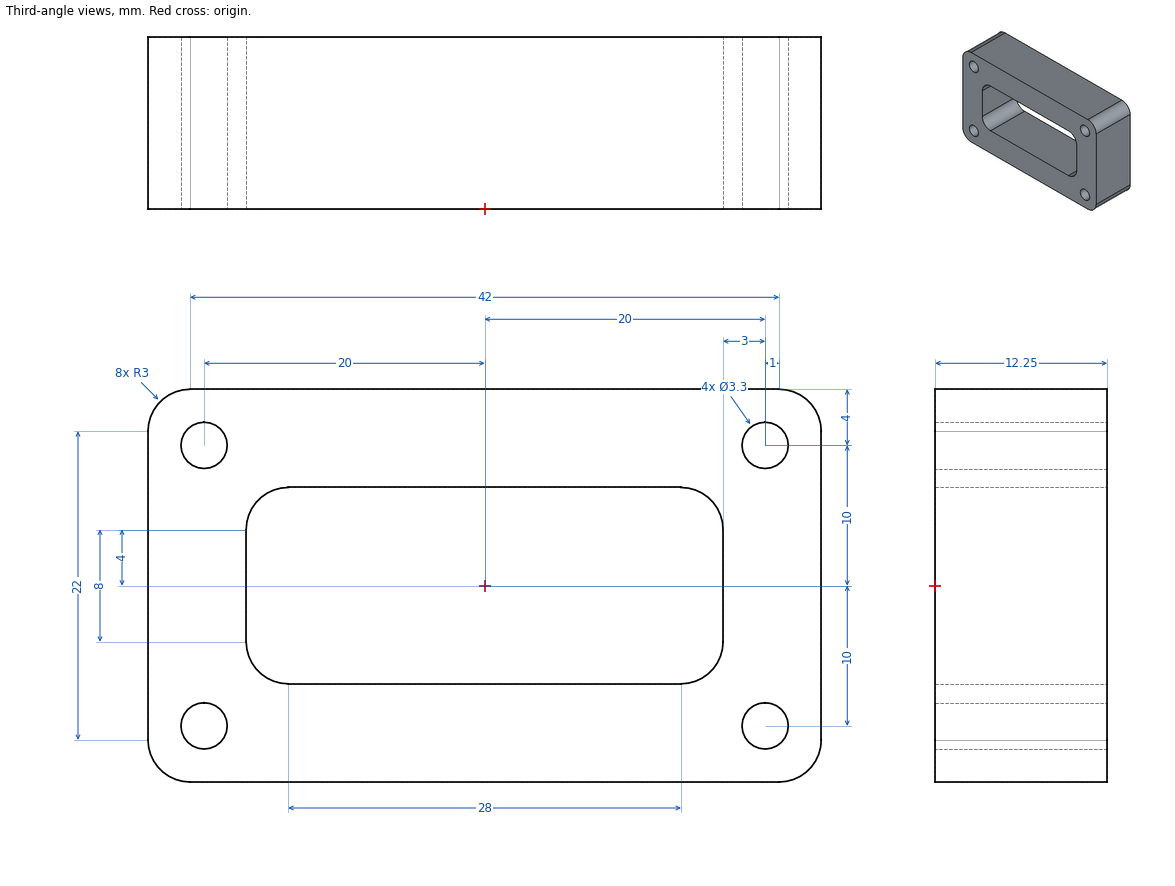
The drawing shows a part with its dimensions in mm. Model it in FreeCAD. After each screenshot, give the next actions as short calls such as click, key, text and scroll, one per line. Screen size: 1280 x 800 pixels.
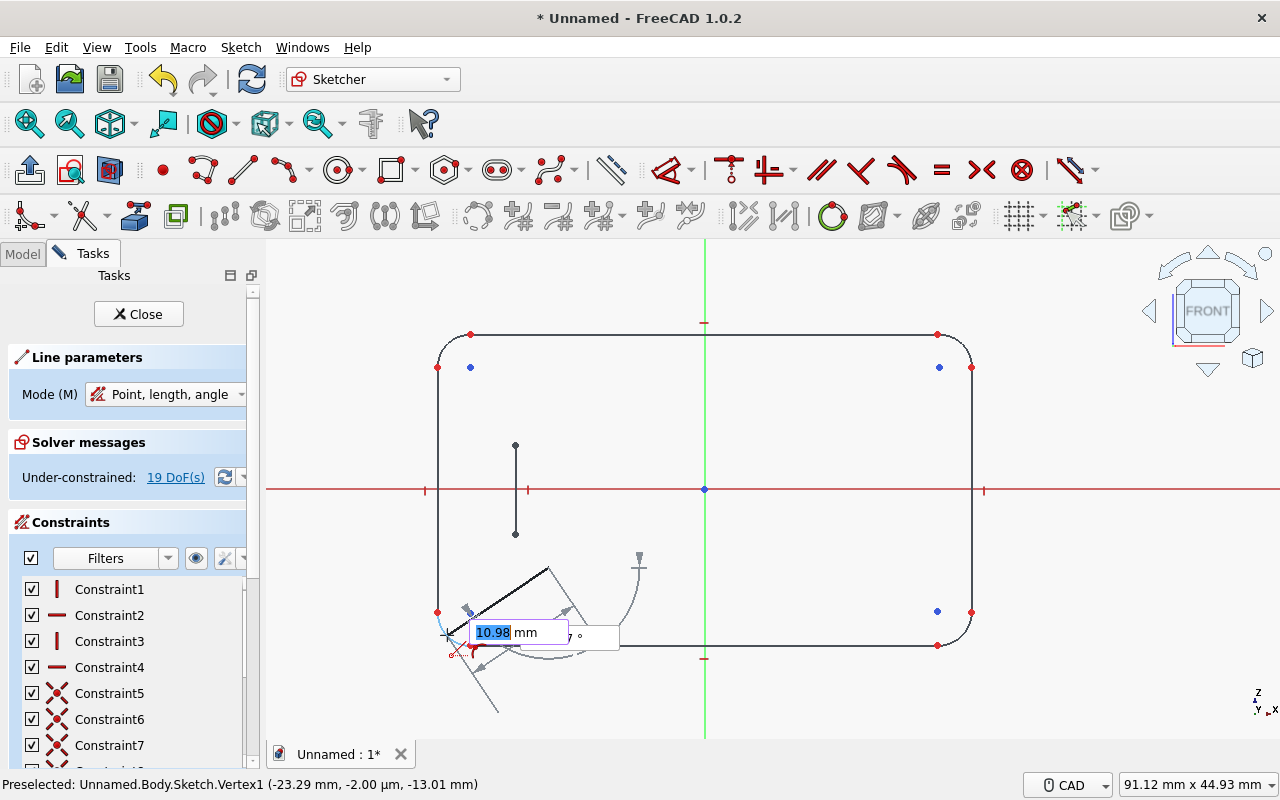
click(860, 567)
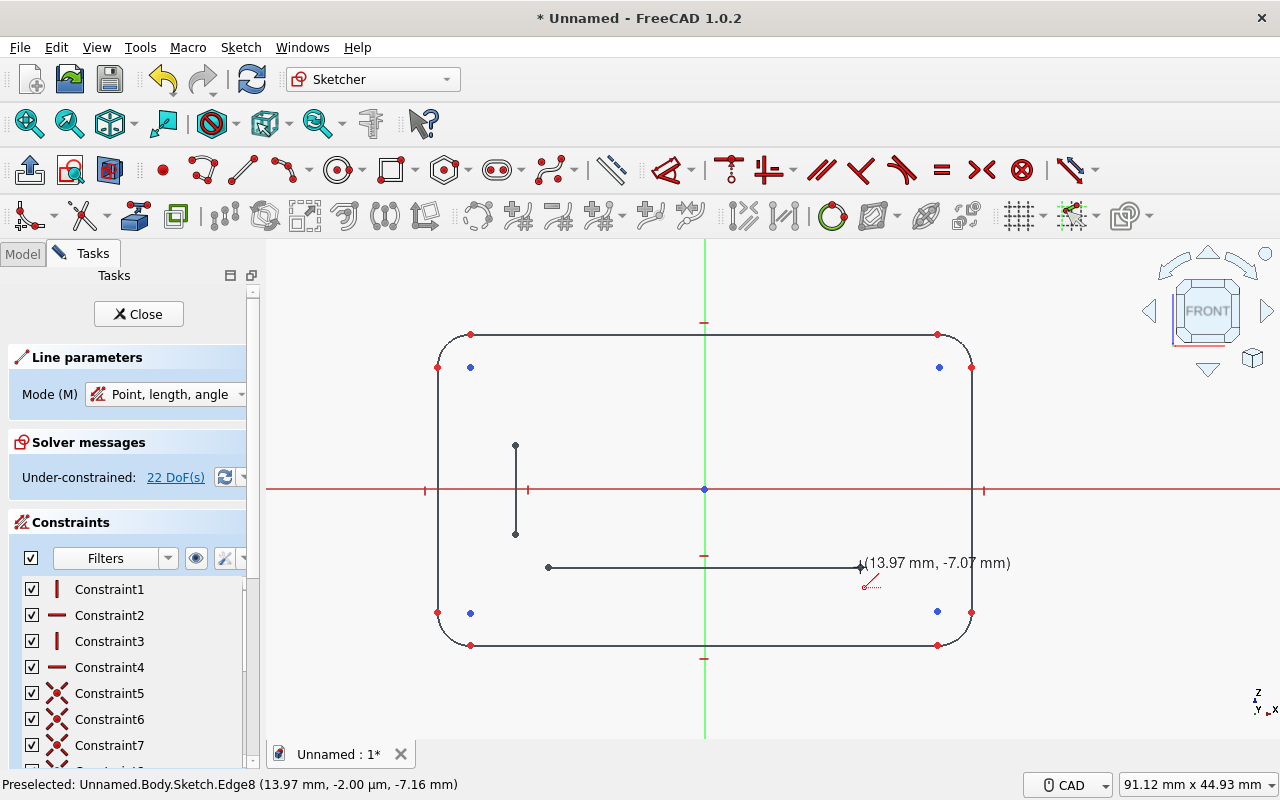
click(894, 534)
click(894, 445)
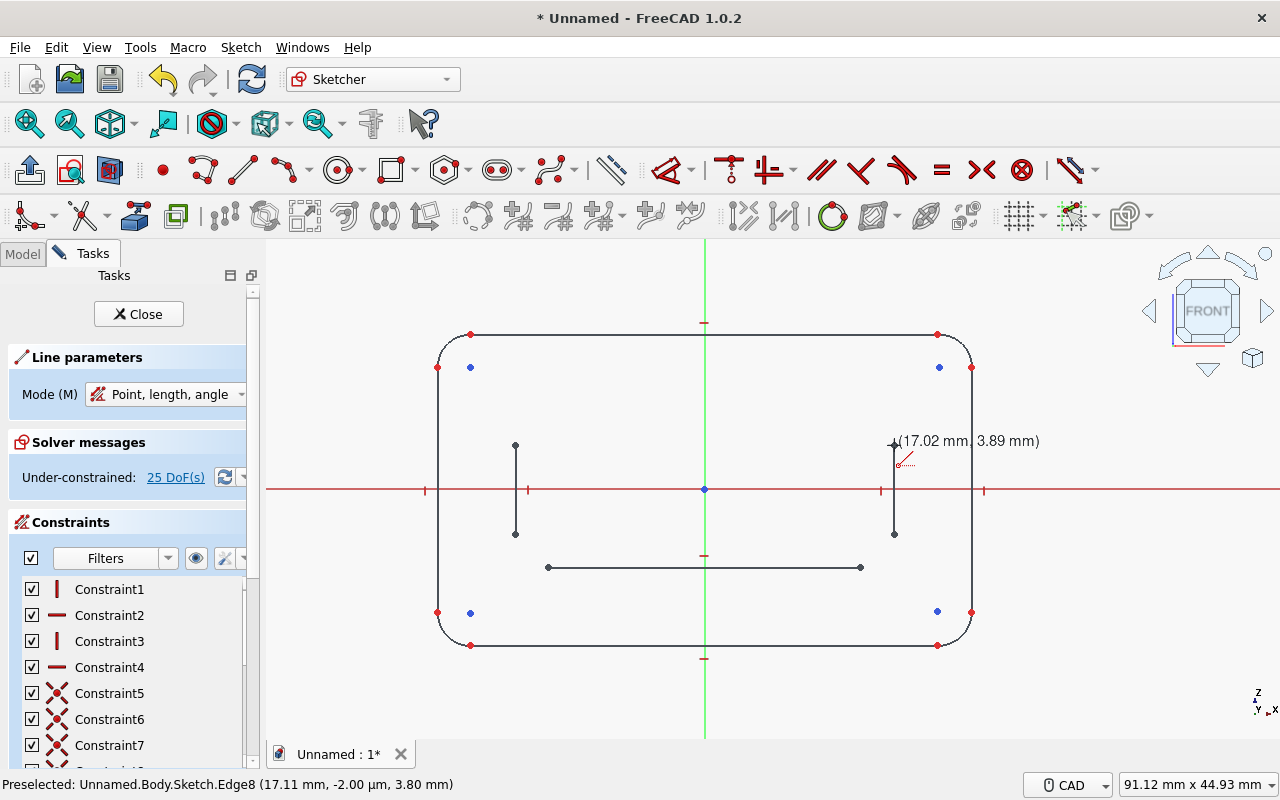
click(860, 411)
click(549, 411)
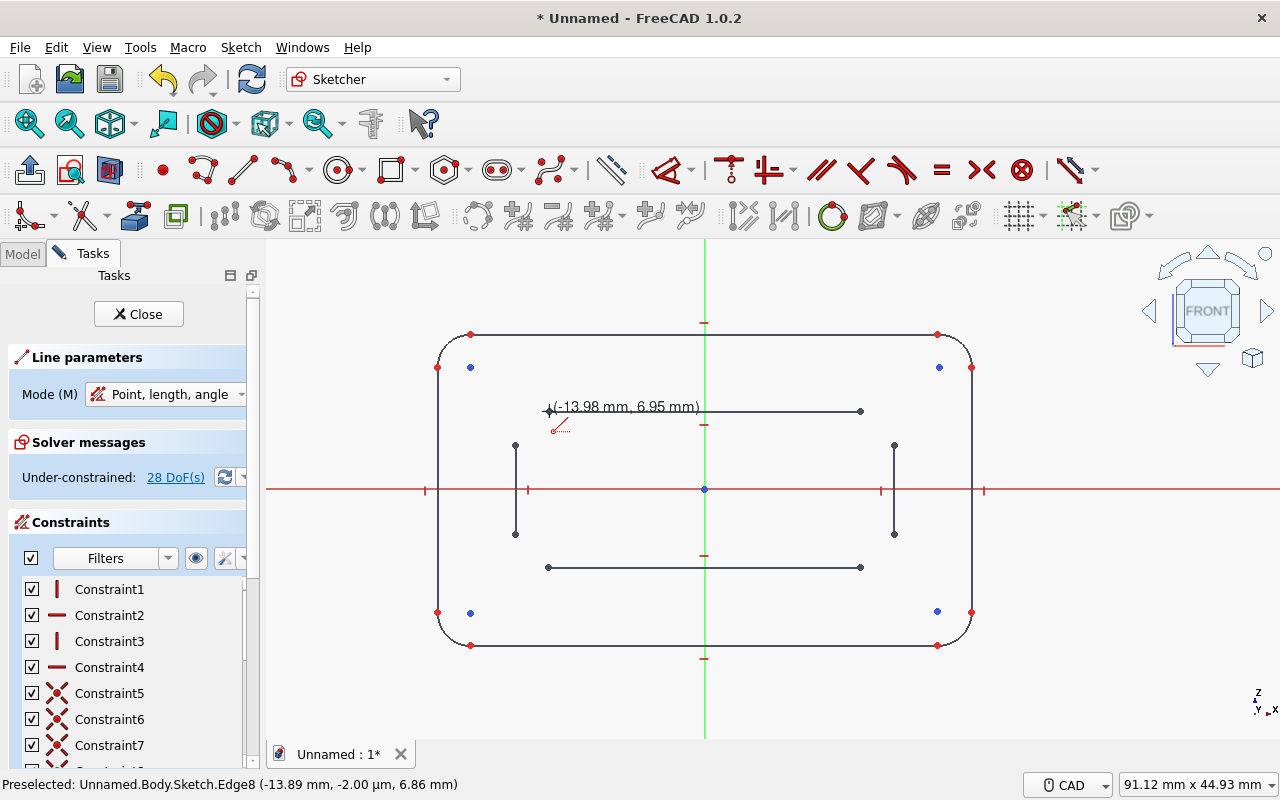
click(284, 170)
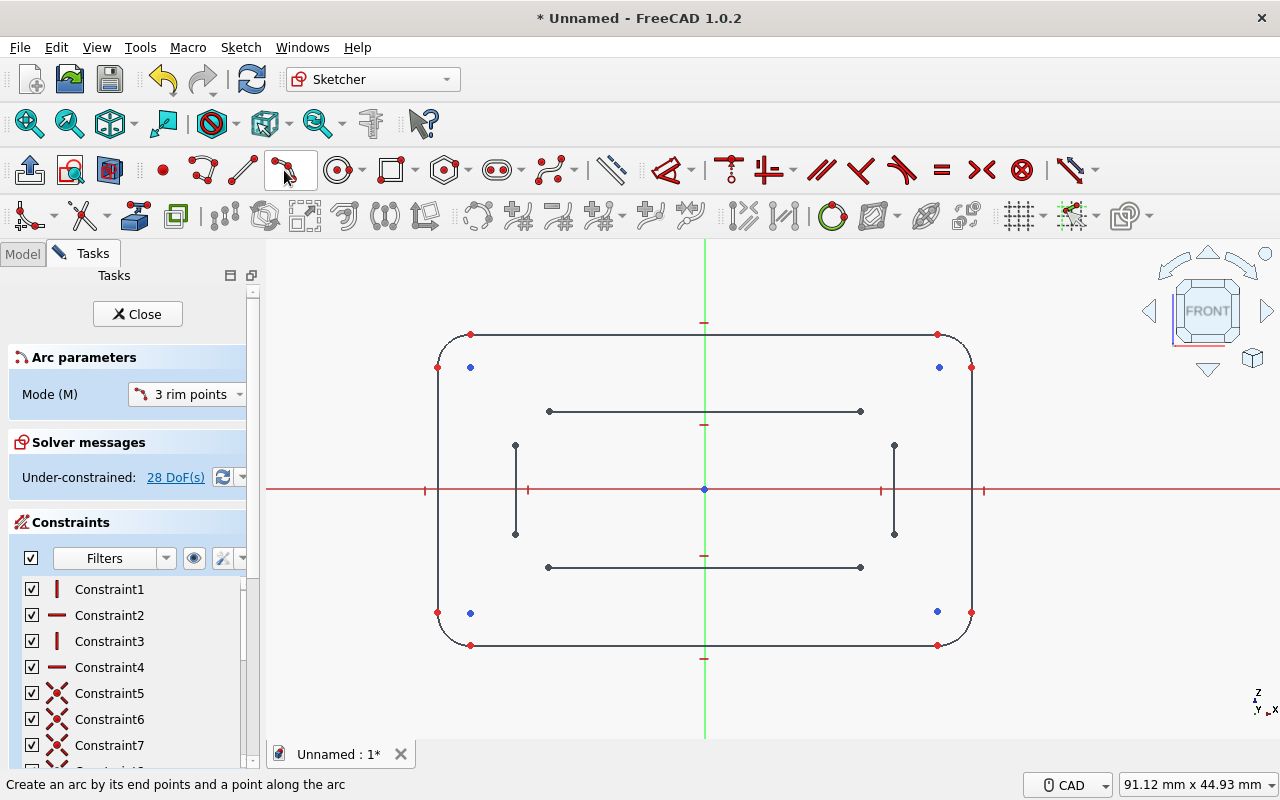
click(516, 534)
click(549, 568)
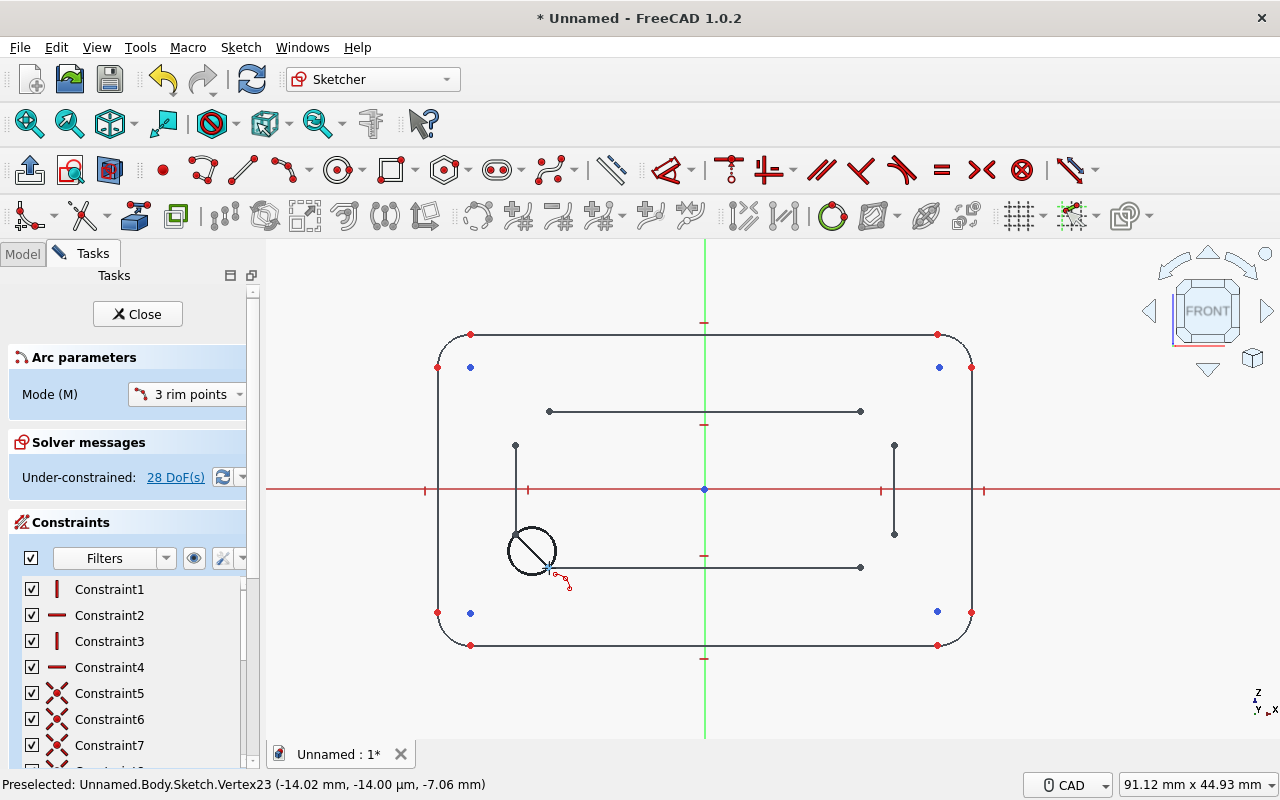
scroll(525, 557, up, 3)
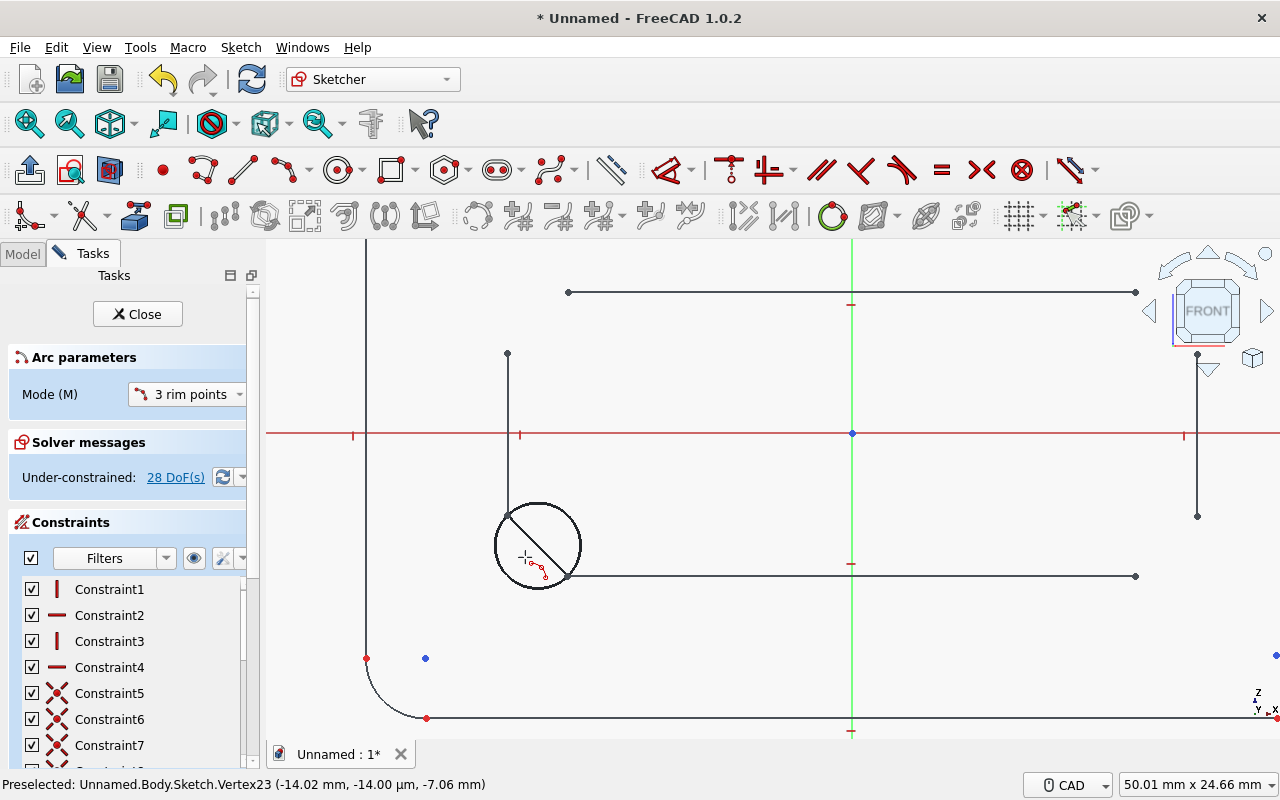
click(525, 557)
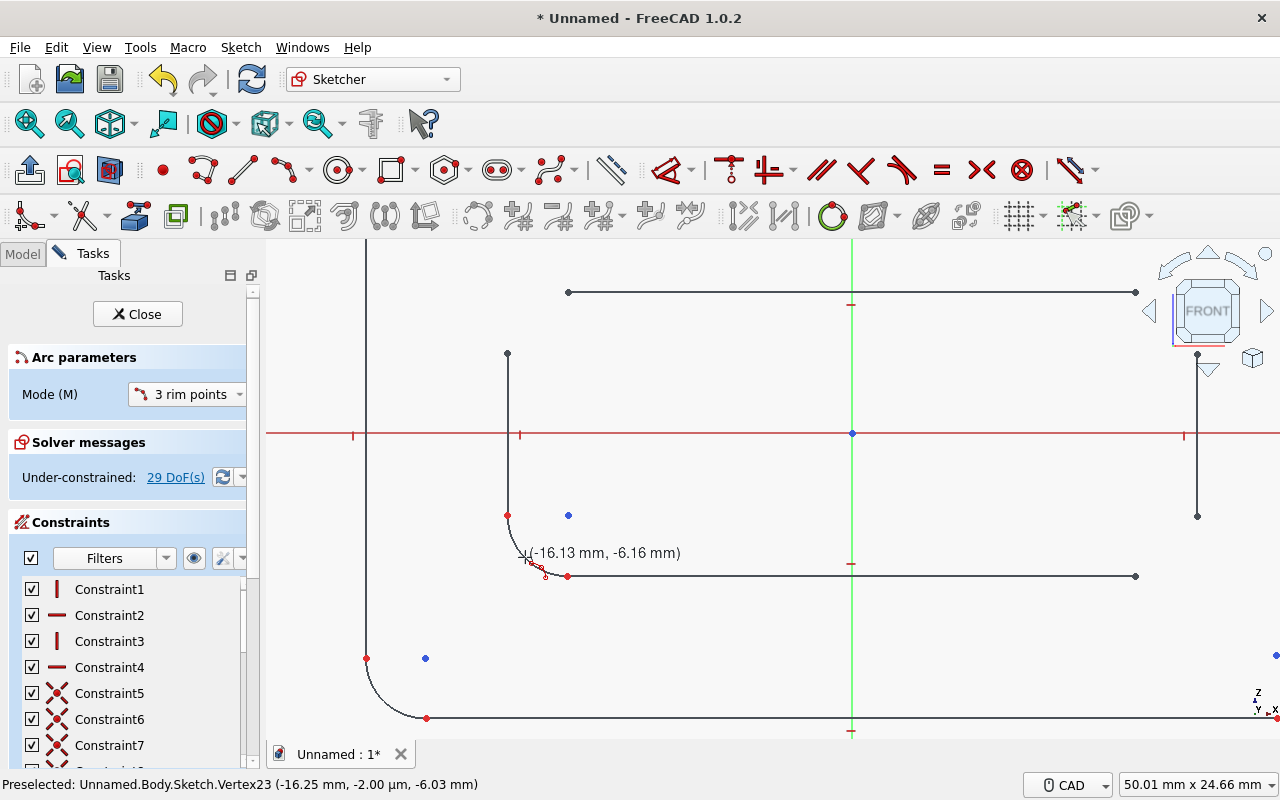
scroll(525, 557, down, 3)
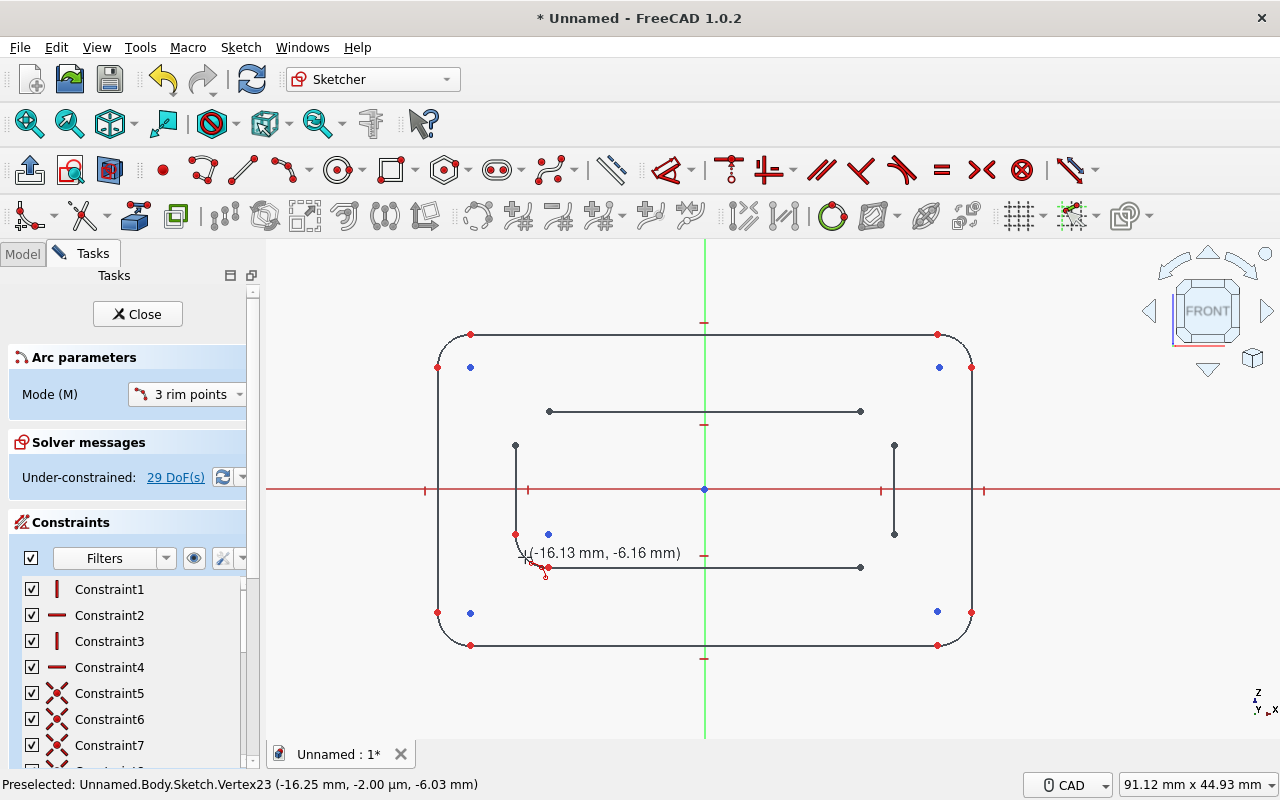
click(860, 568)
click(894, 535)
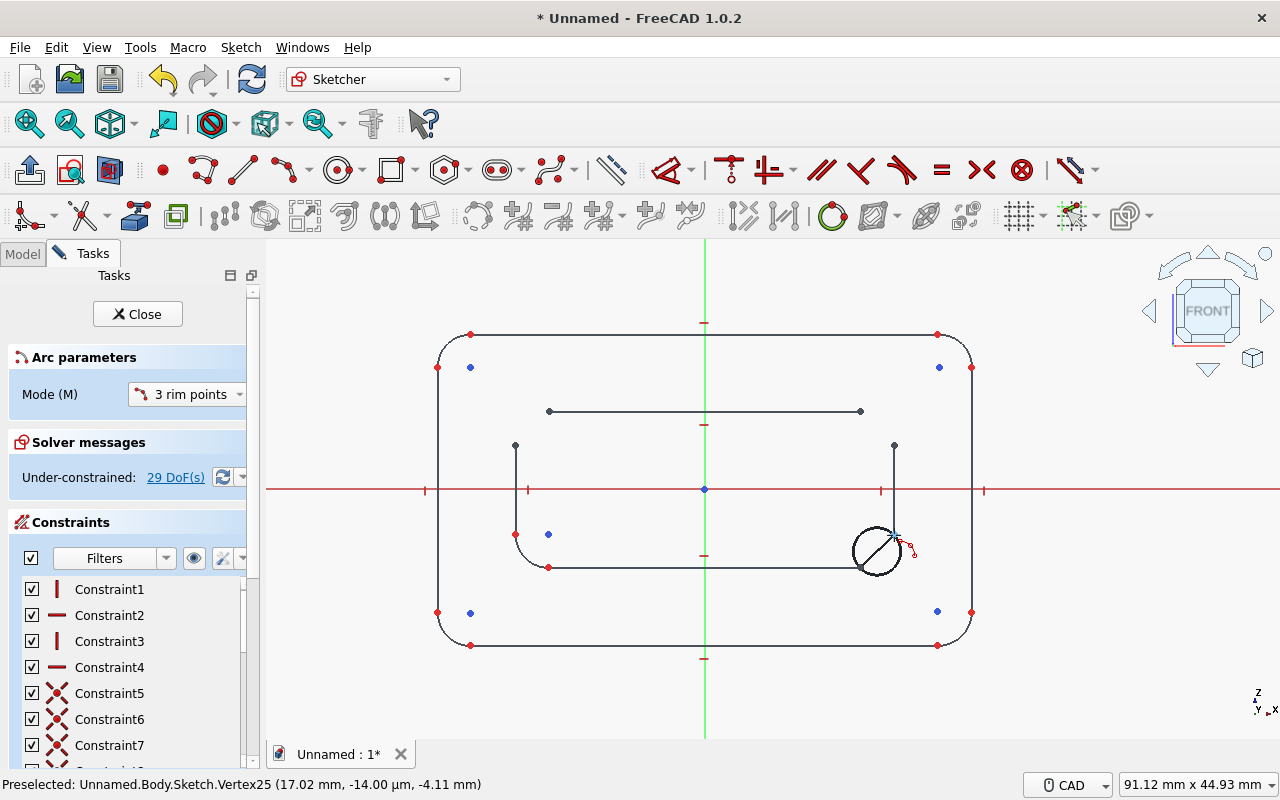
scroll(884, 557, up, 3)